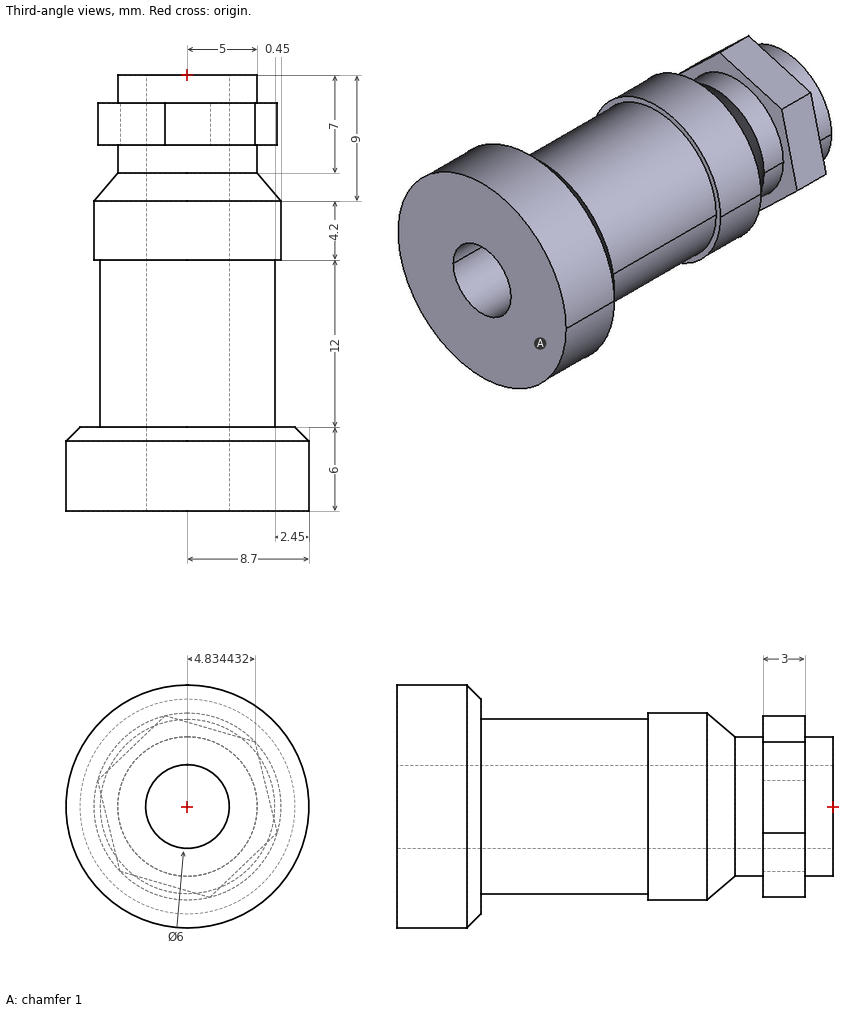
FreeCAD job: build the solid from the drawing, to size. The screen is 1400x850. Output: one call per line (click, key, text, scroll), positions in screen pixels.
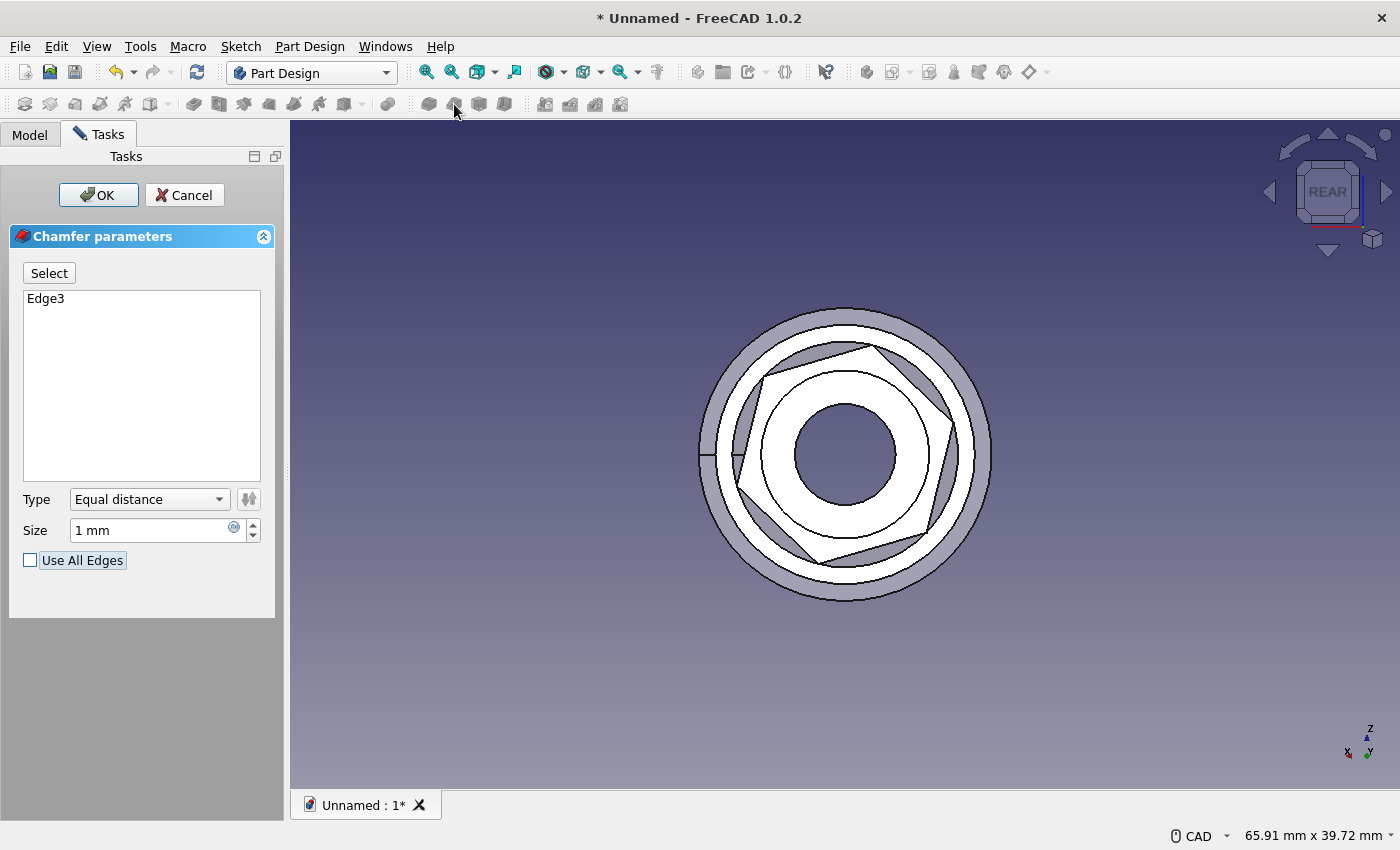
click(99, 195)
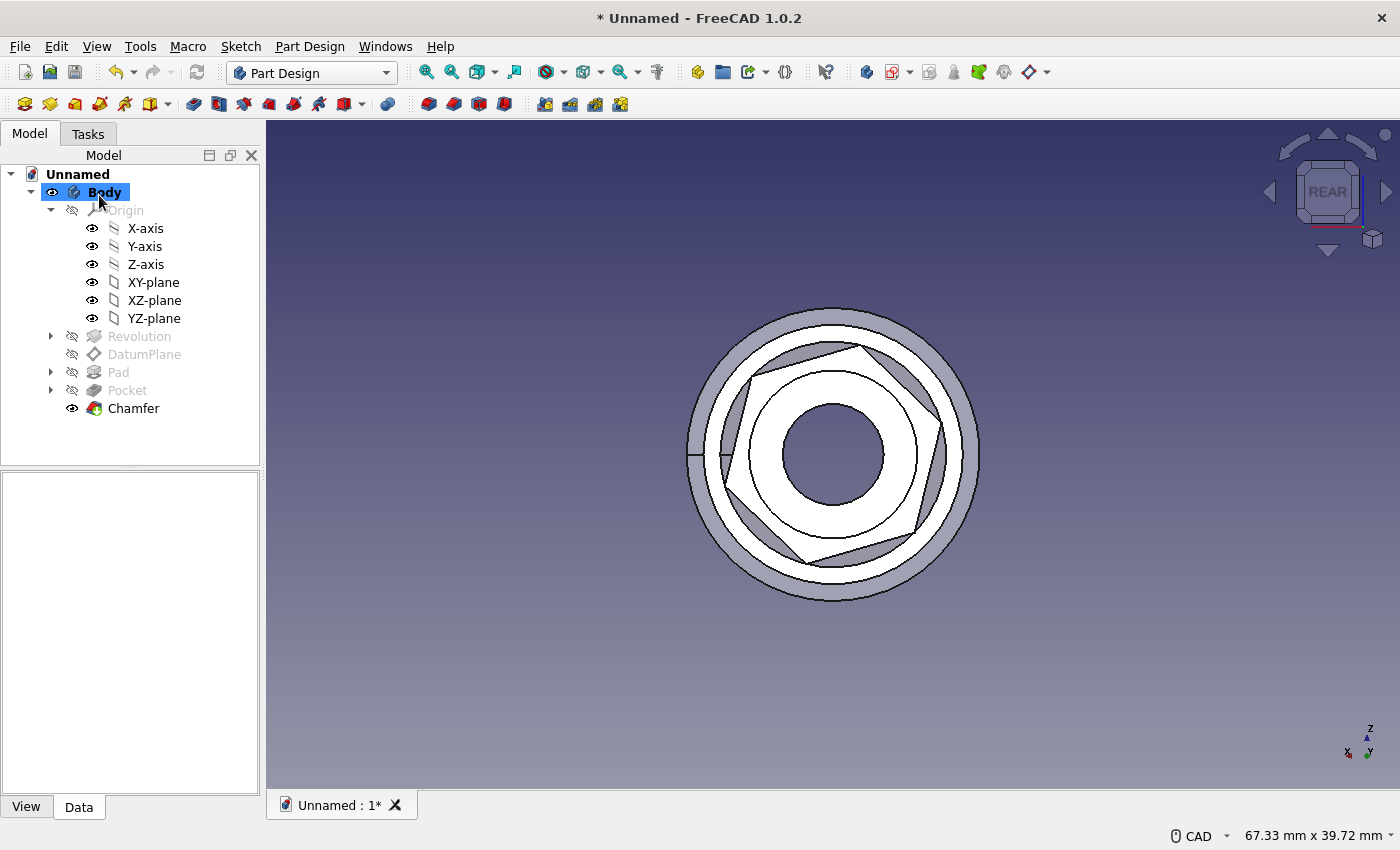
key(0)